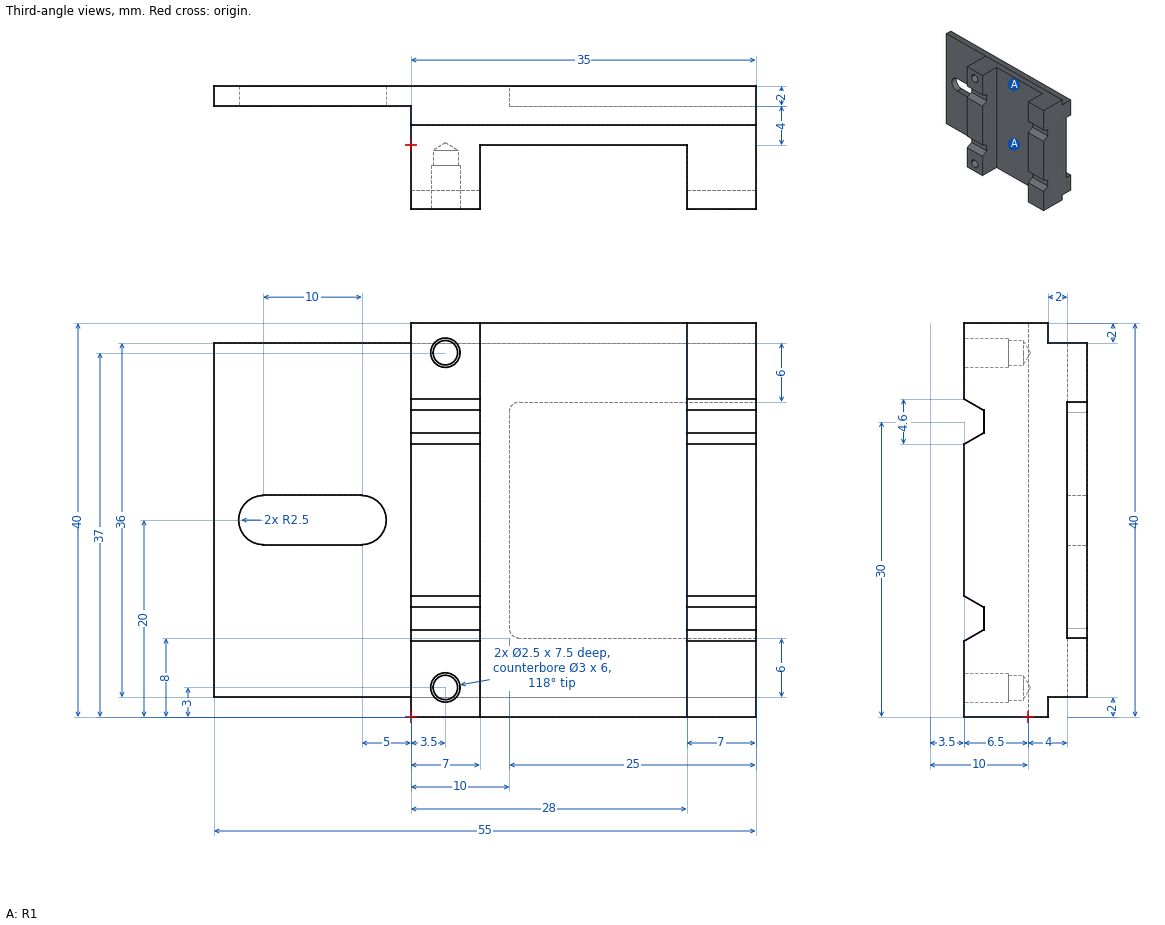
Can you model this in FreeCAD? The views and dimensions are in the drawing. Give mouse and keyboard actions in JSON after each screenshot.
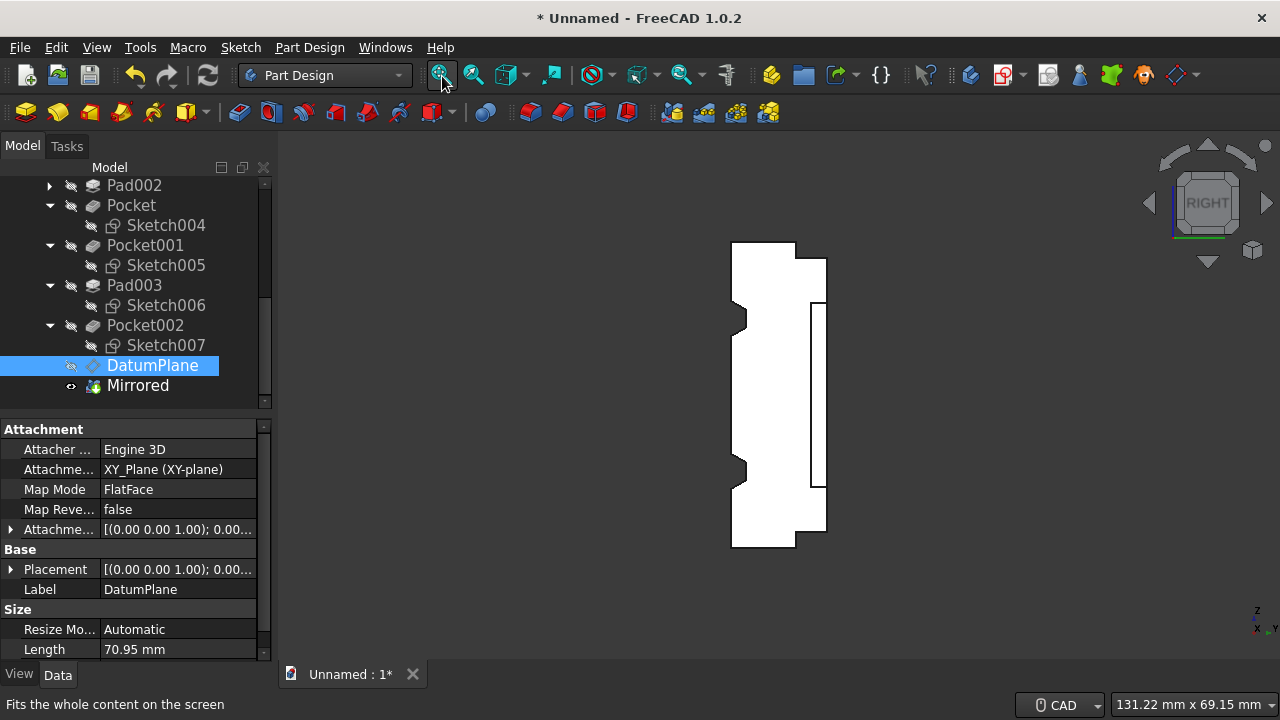
{"action": "scroll", "coordinate": [819, 302], "scroll_direction": "up", "scroll_amount": 5}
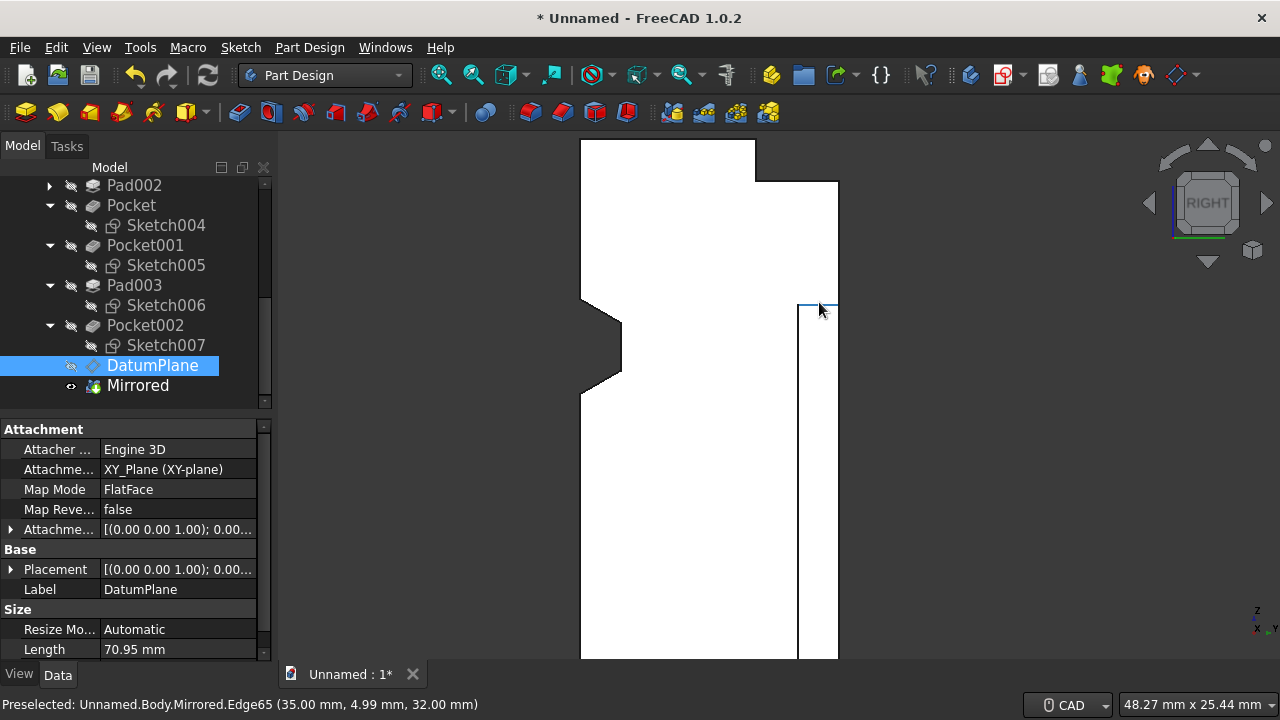
{"action": "left_click", "coordinate": [442, 76]}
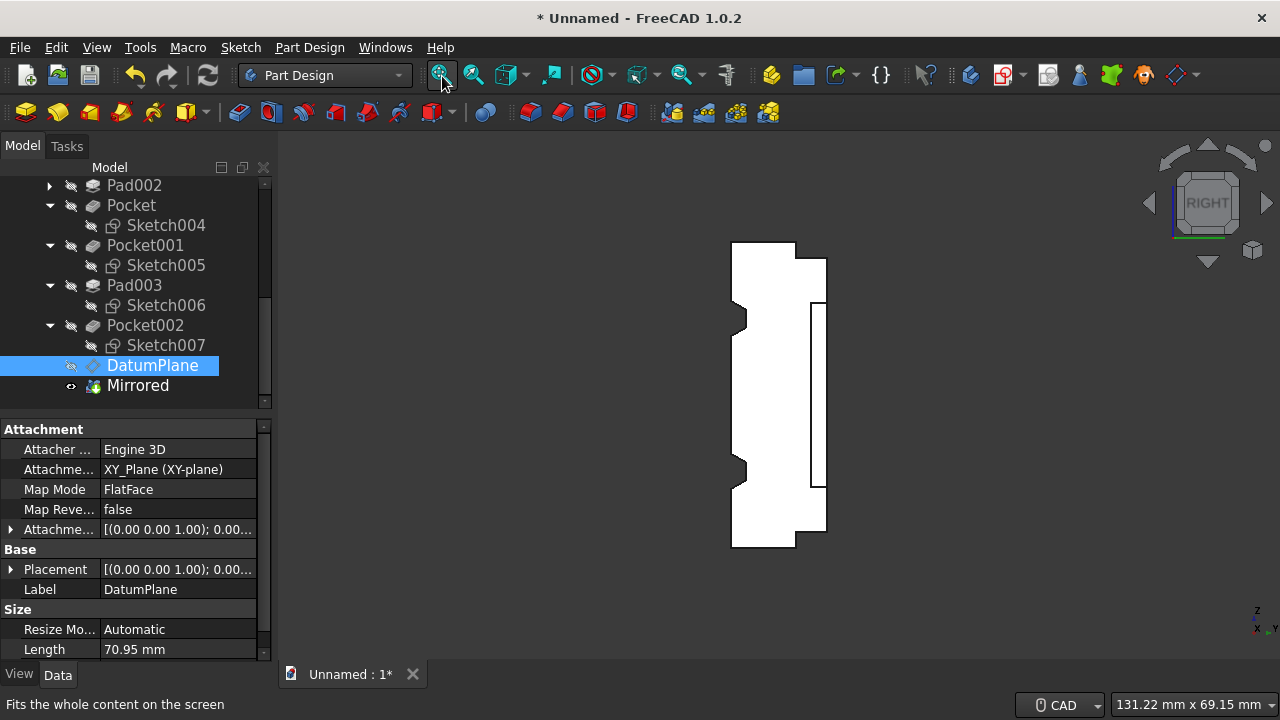
{"action": "key", "text": "5"}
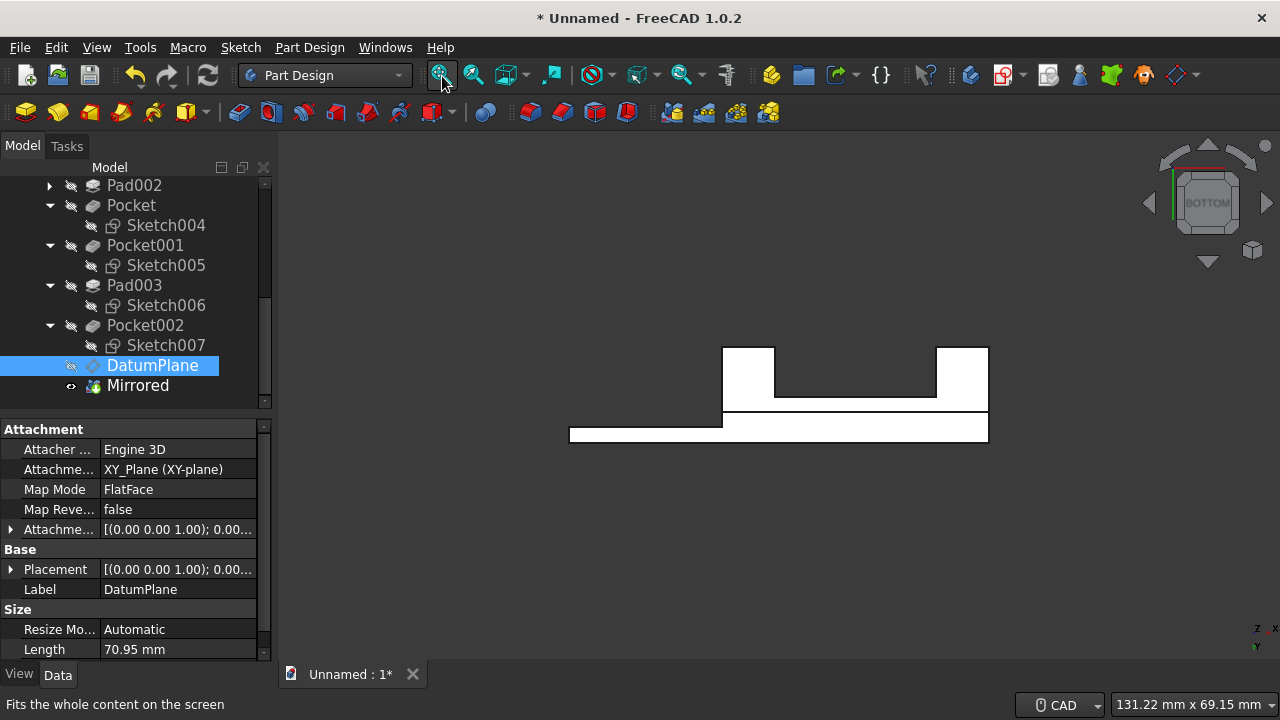
{"action": "left_click", "coordinate": [442, 76]}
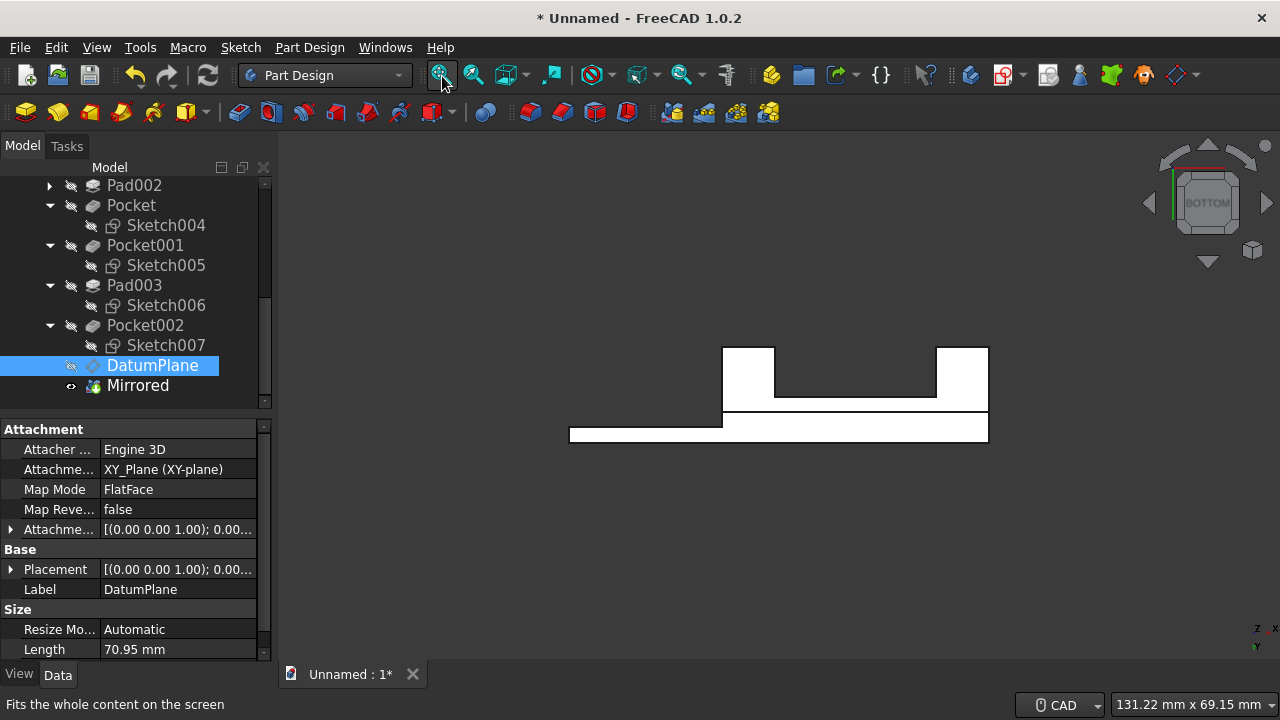
{"action": "scroll", "coordinate": [798, 434], "scroll_direction": "up", "scroll_amount": 5}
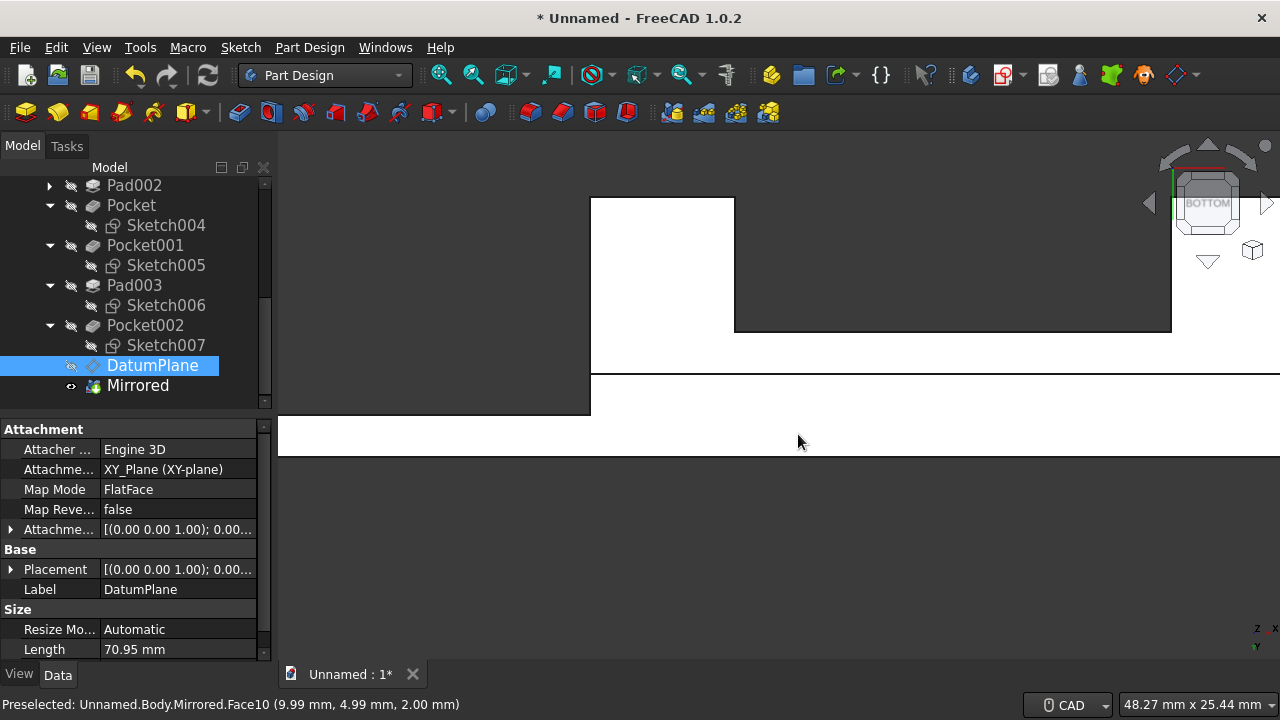
{"action": "left_click", "coordinate": [442, 76]}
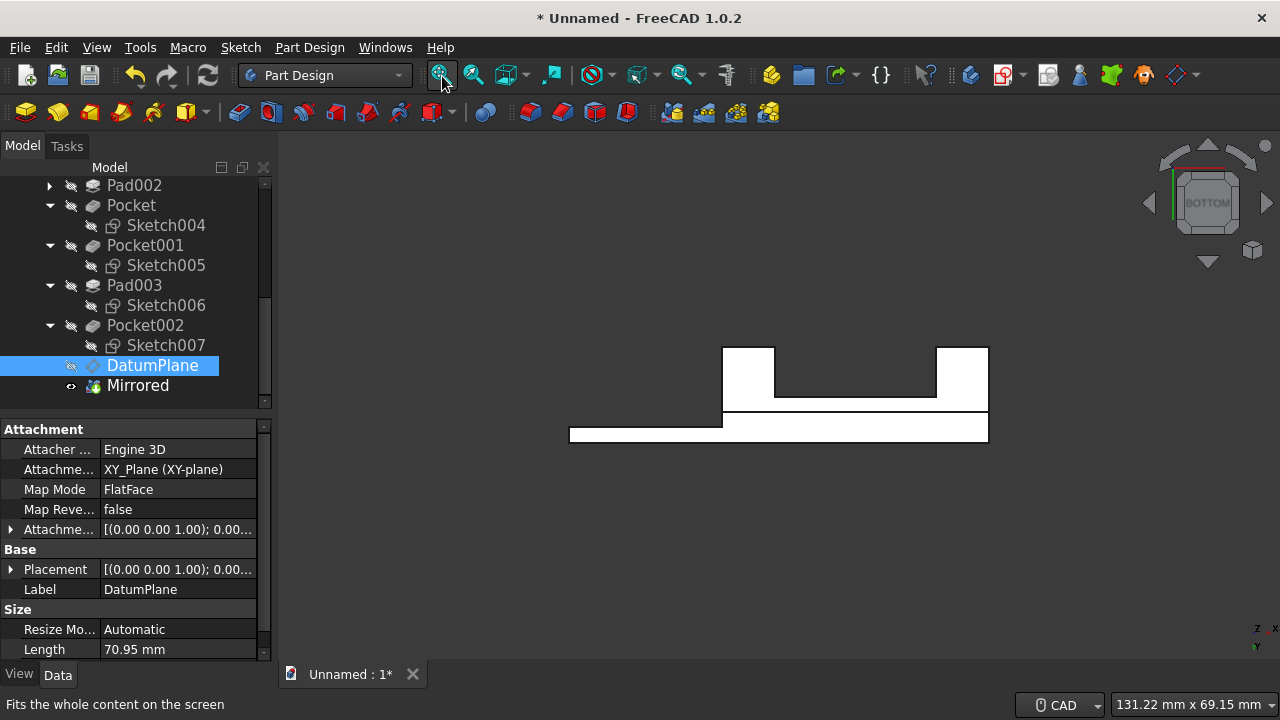
{"action": "key", "text": "4"}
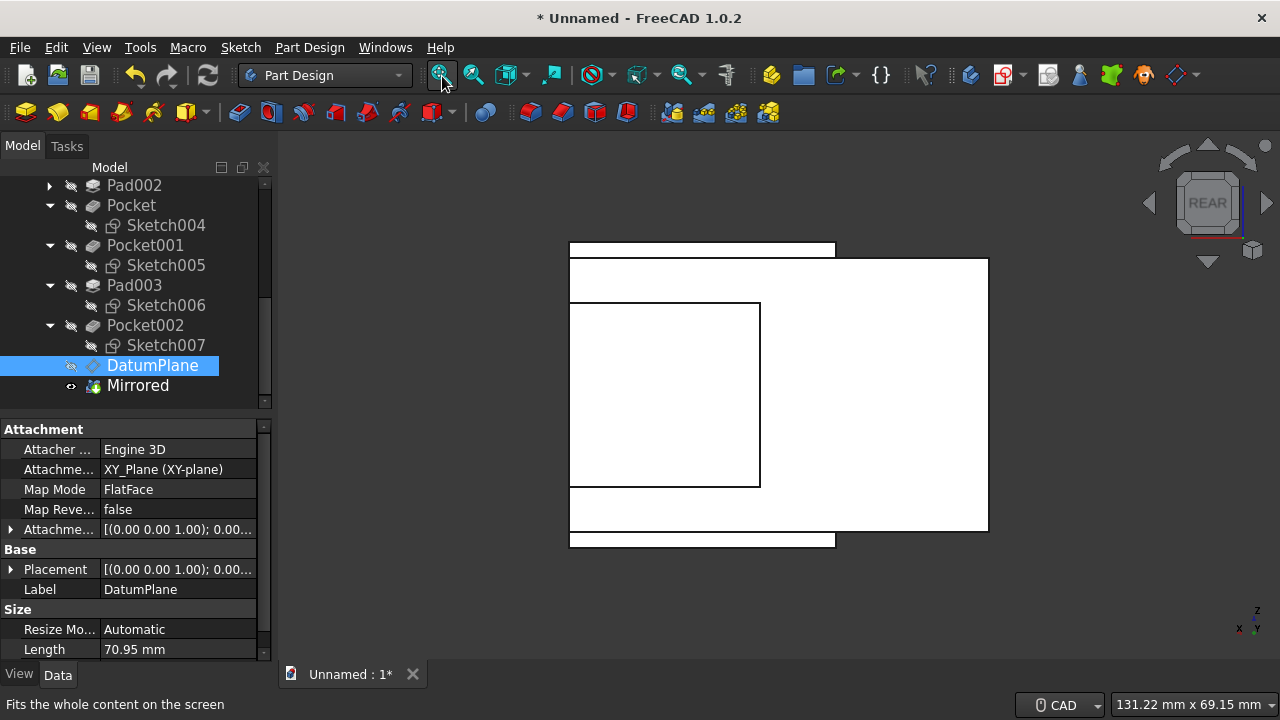
{"action": "scroll", "coordinate": [760, 302], "scroll_direction": "up", "scroll_amount": 5}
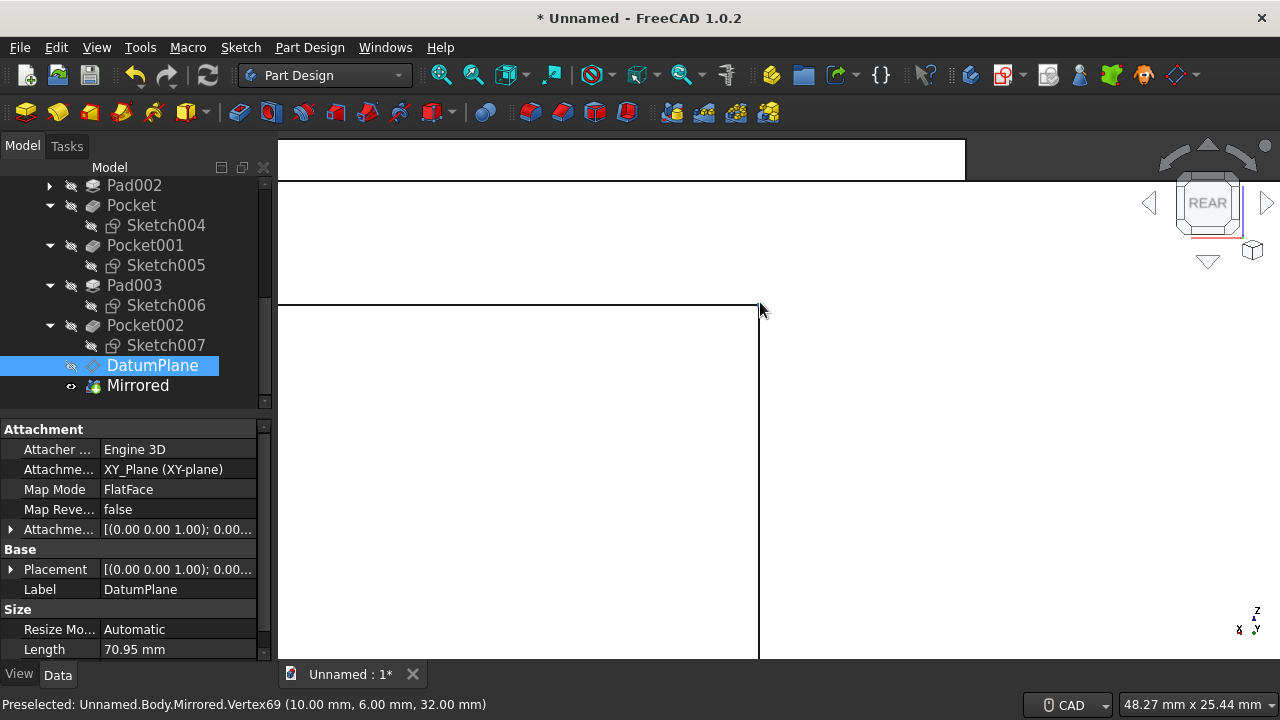
{"action": "left_click", "coordinate": [442, 76]}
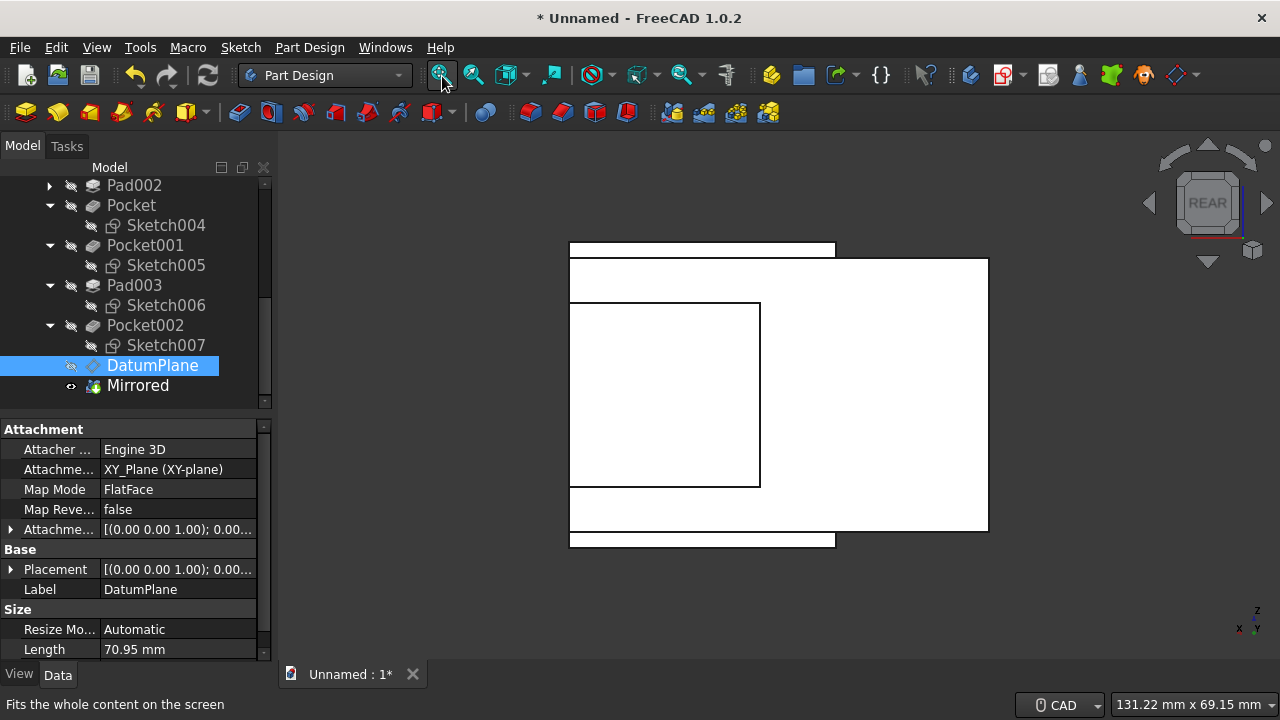
{"action": "key", "text": "6"}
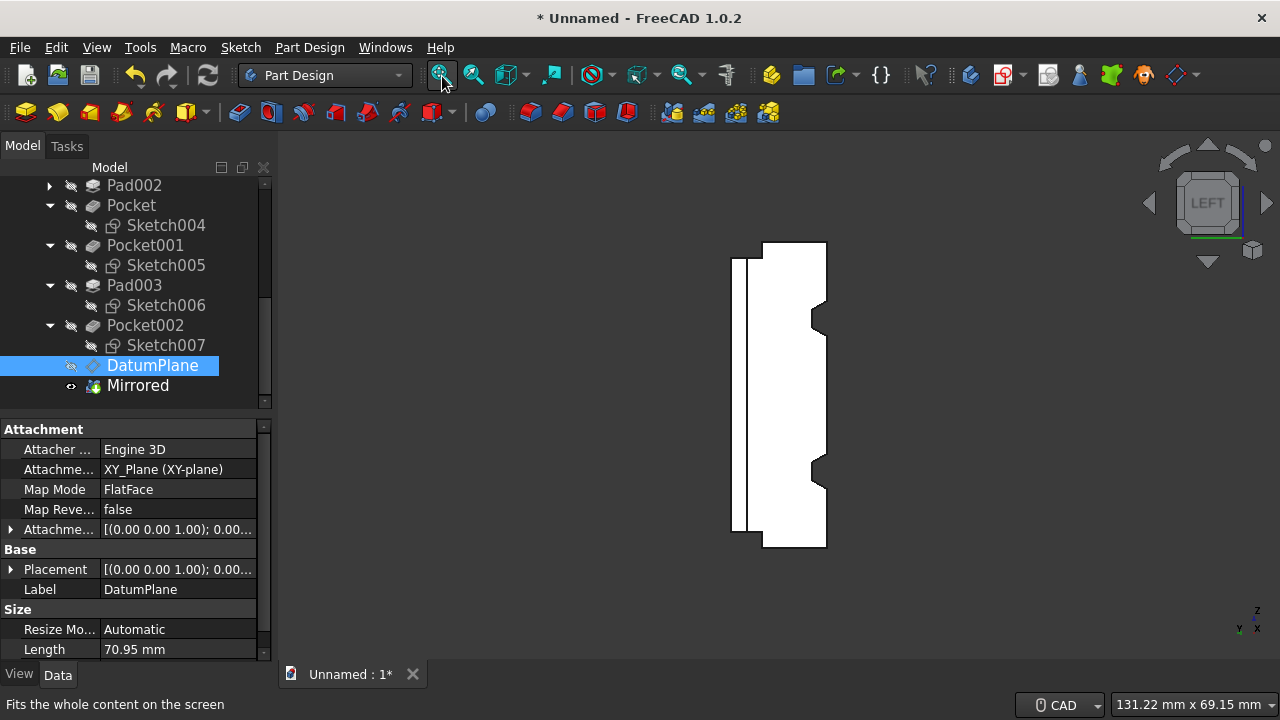
{"action": "scroll", "coordinate": [739, 302], "scroll_direction": "up", "scroll_amount": 5}